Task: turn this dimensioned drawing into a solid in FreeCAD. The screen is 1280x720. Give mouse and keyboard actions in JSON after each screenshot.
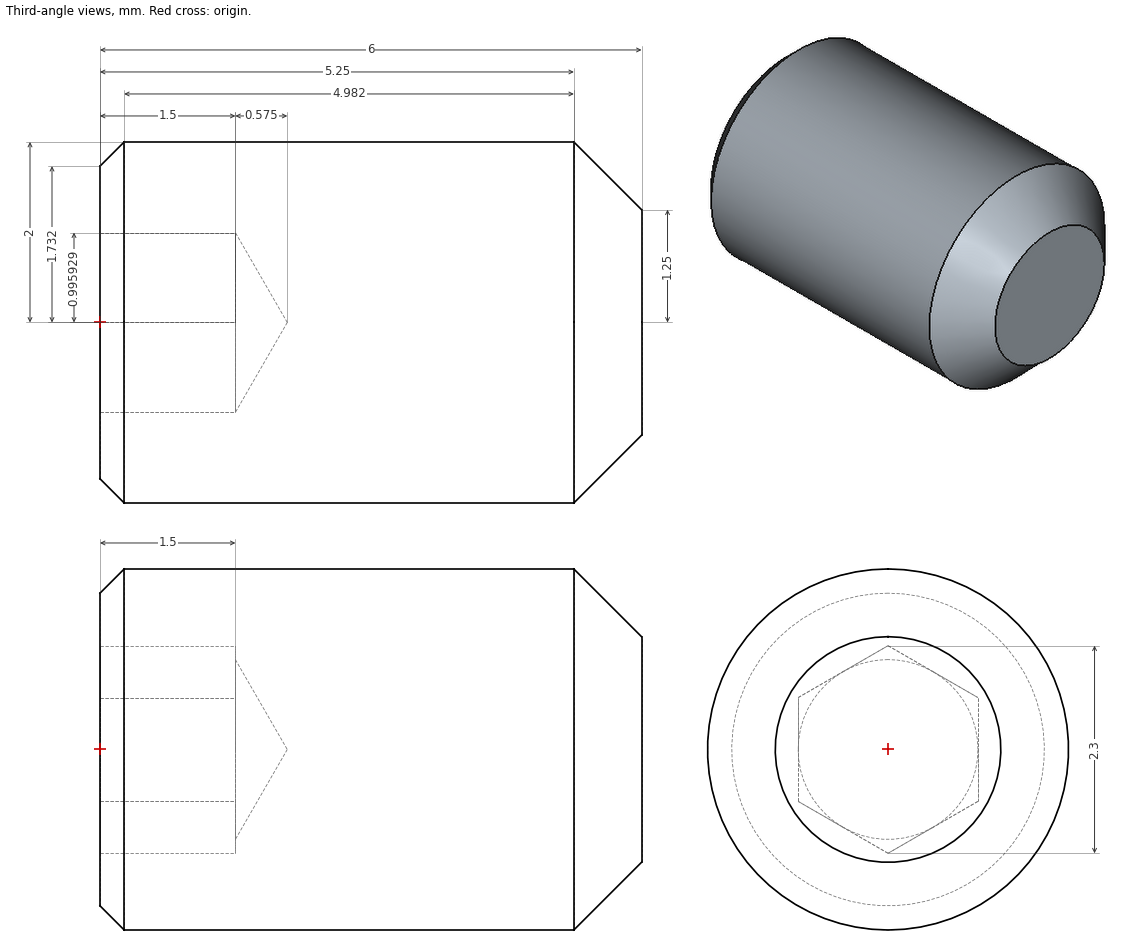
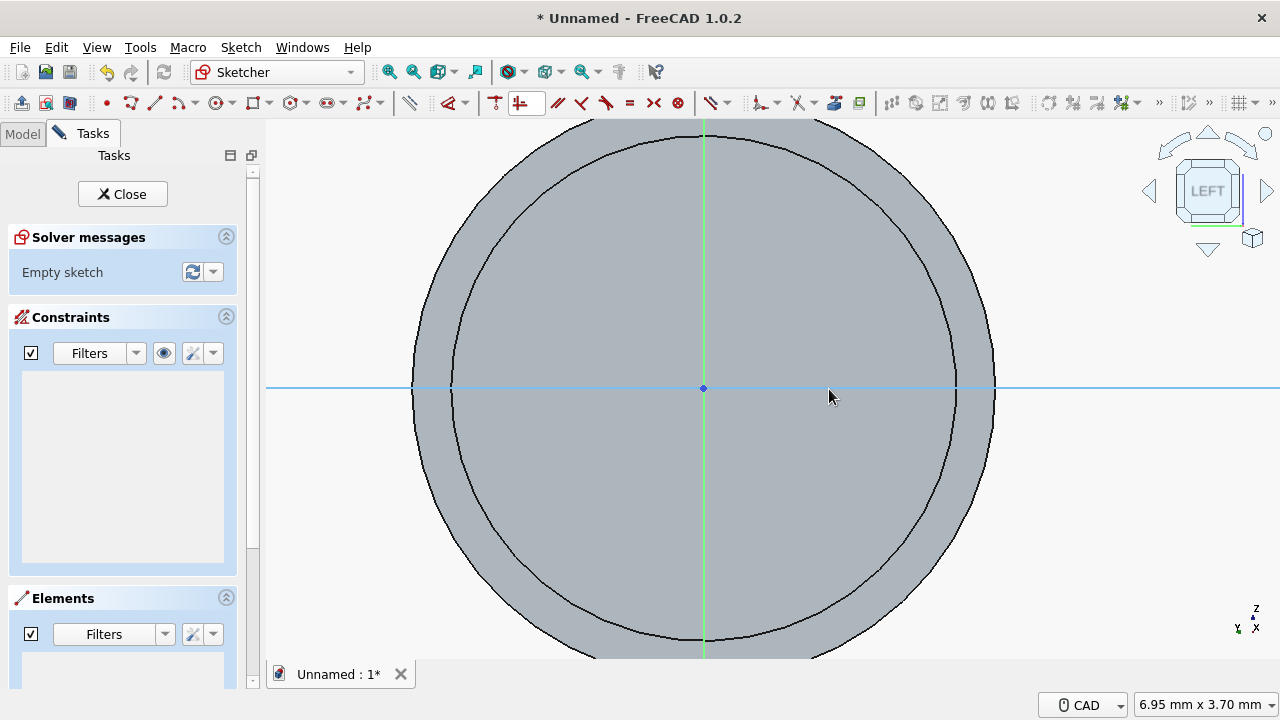
{"action": "left_click", "coordinate": [290, 104]}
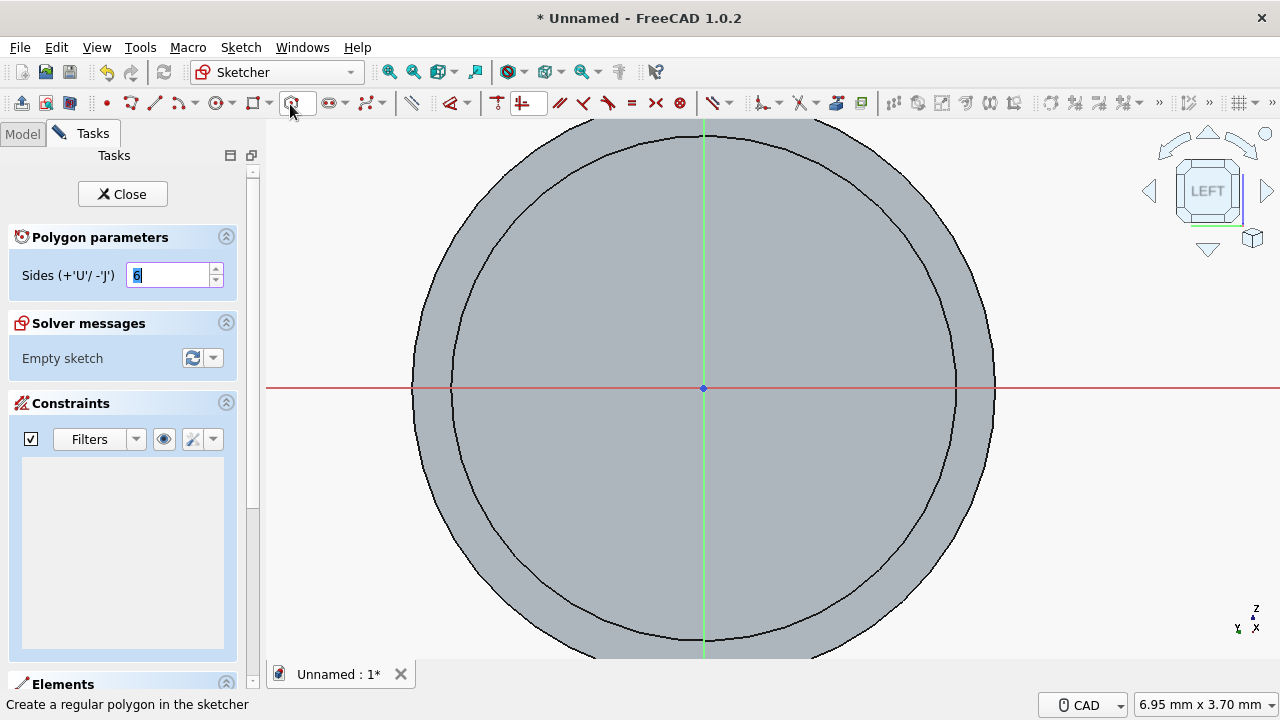
{"action": "left_click", "coordinate": [704, 388]}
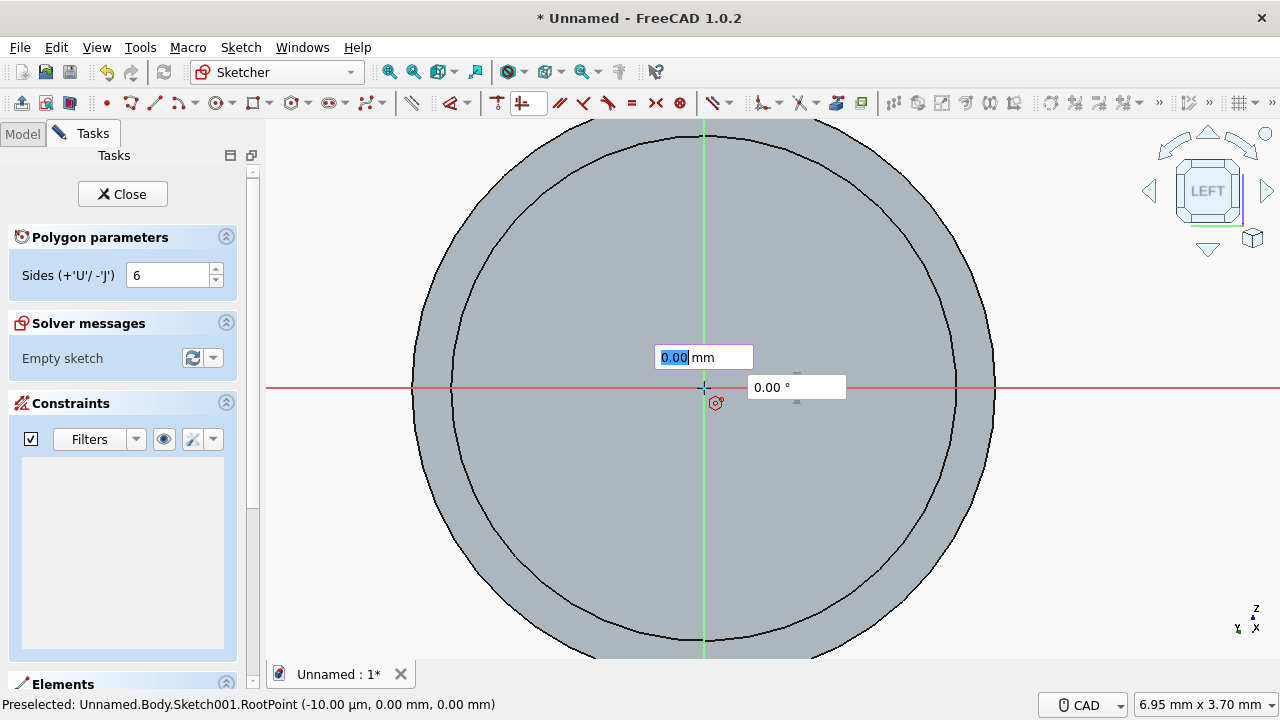
{"action": "left_click", "coordinate": [704, 221]}
{"action": "right_click", "coordinate": [704, 221]}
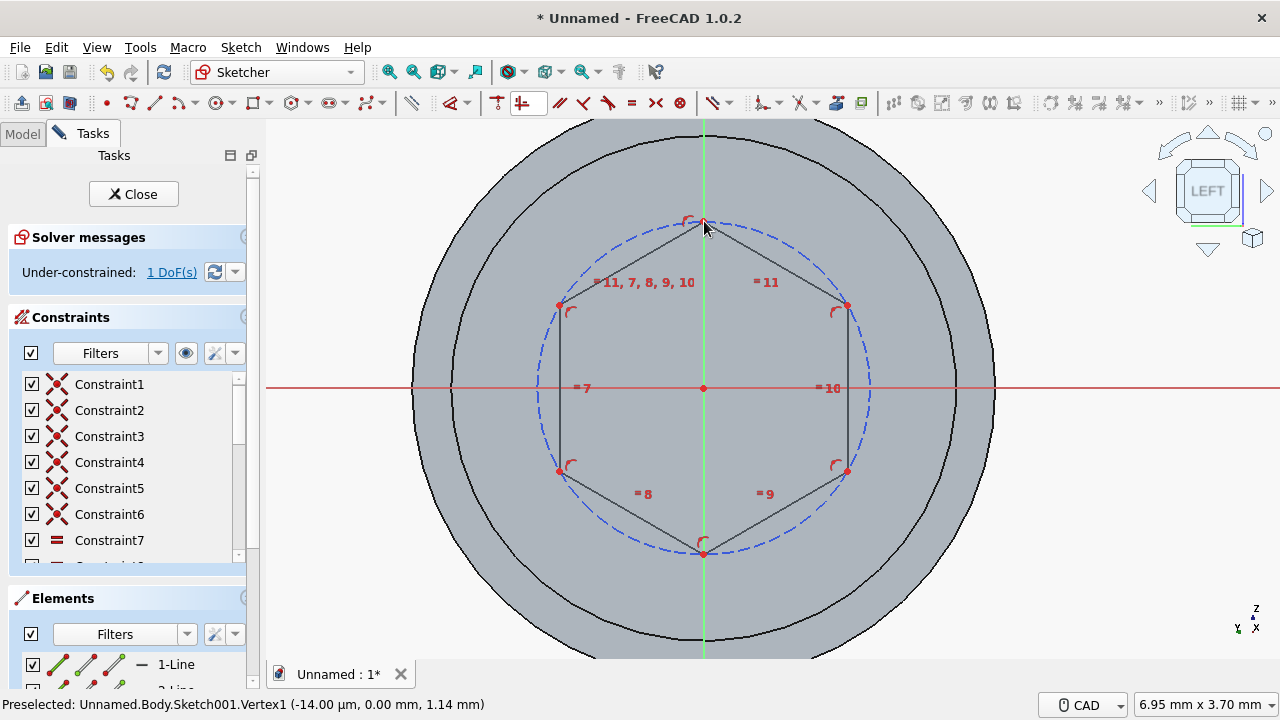
{"action": "left_click", "coordinate": [450, 104]}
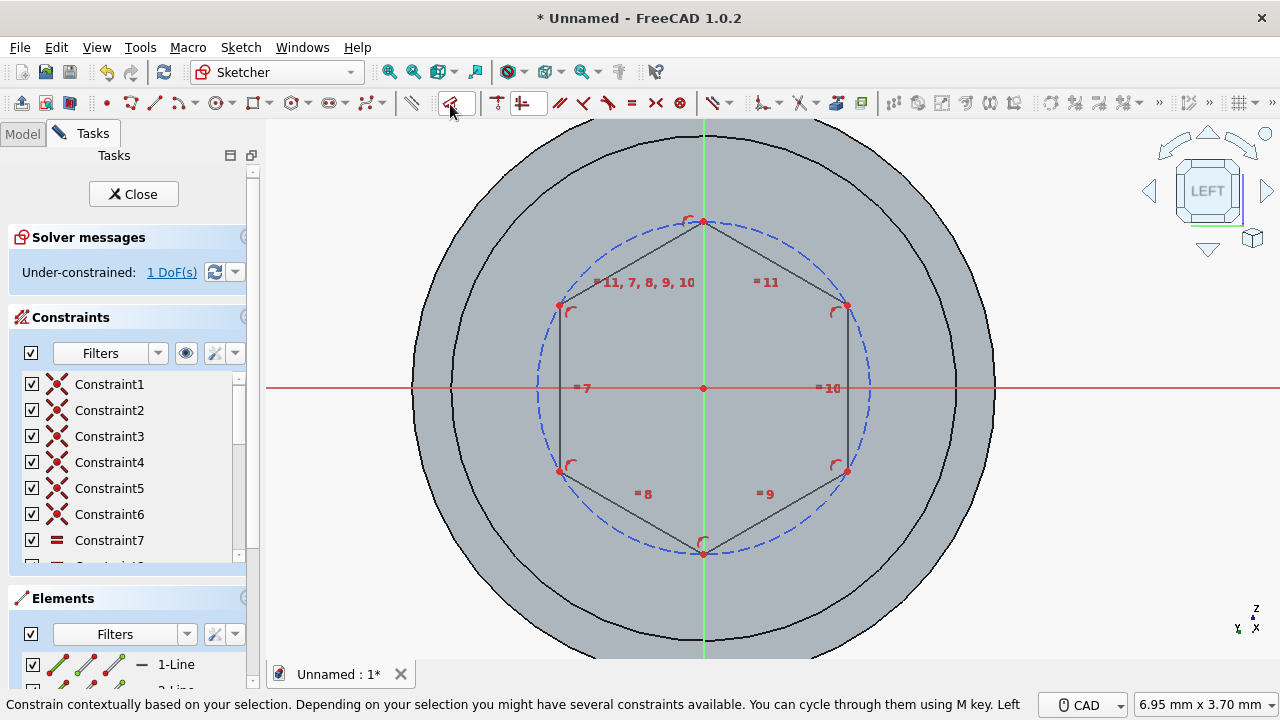
{"action": "left_click", "coordinate": [704, 555]}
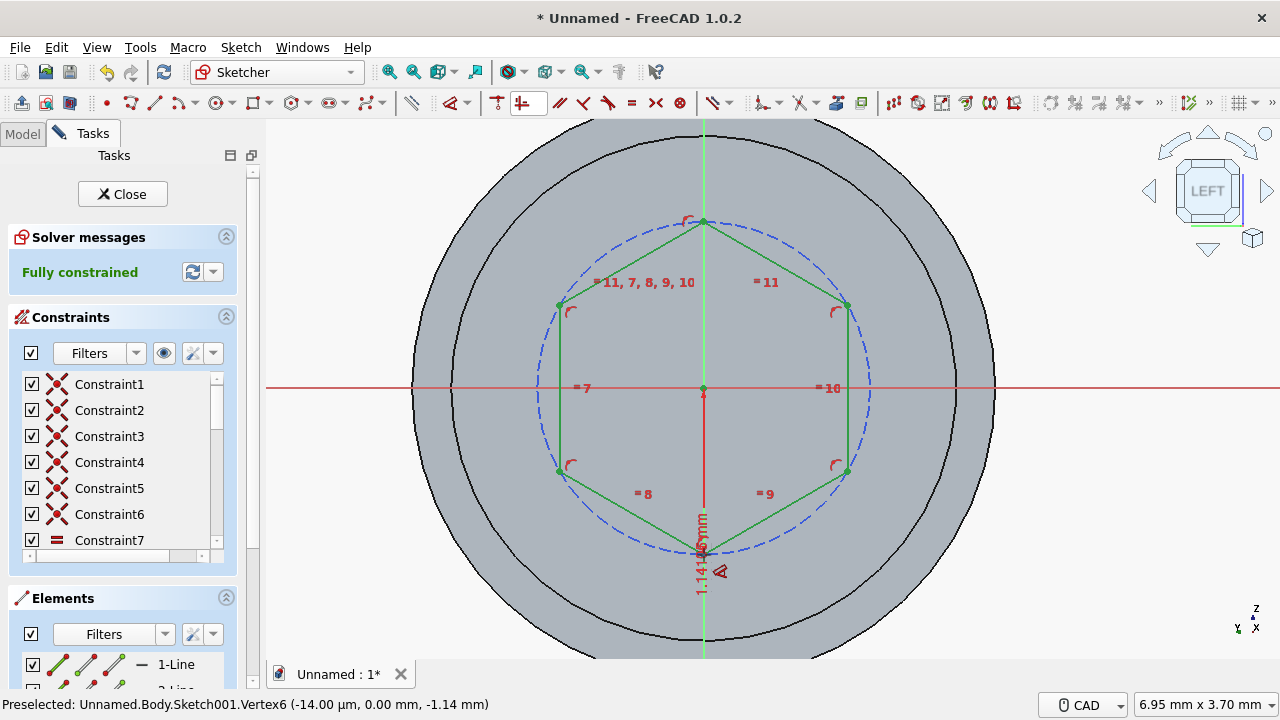
{"action": "left_click", "coordinate": [704, 222]}
{"action": "left_click", "coordinate": [738, 312]}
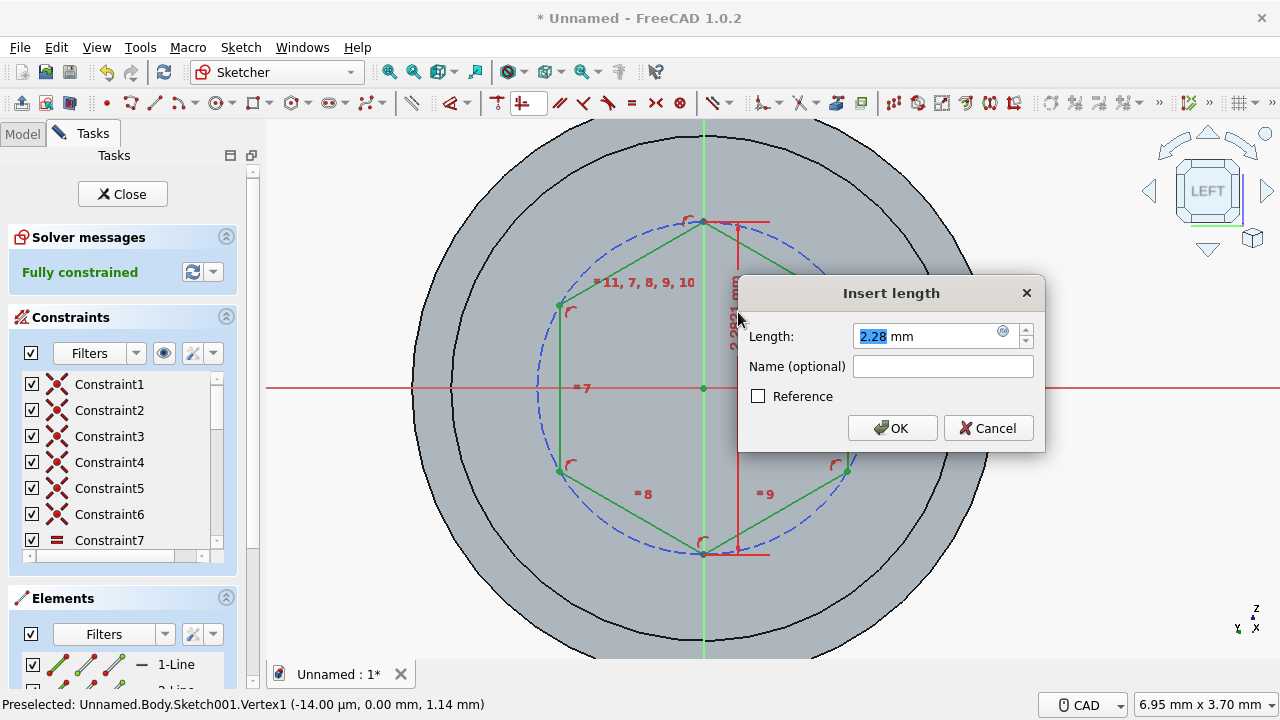
{"action": "type", "text": "2.3"}
{"action": "key", "text": "Return"}
{"action": "key", "text": "Escape"}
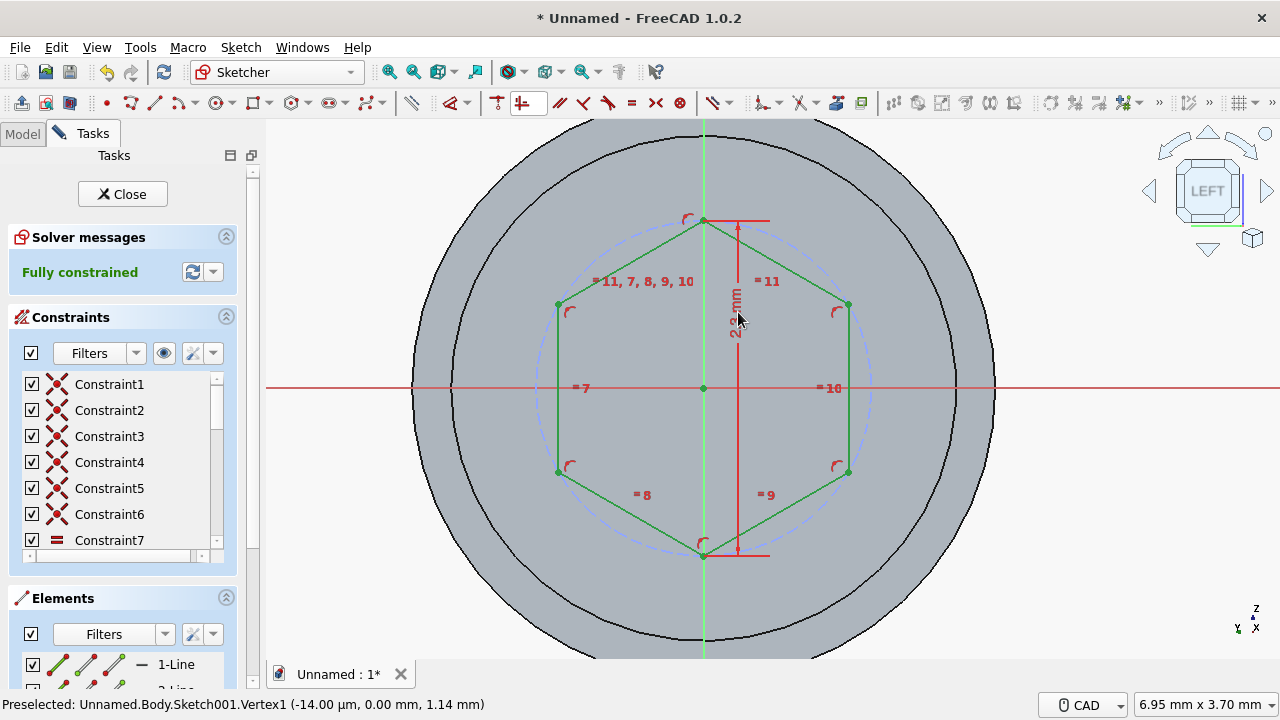
{"action": "left_click", "coordinate": [123, 194]}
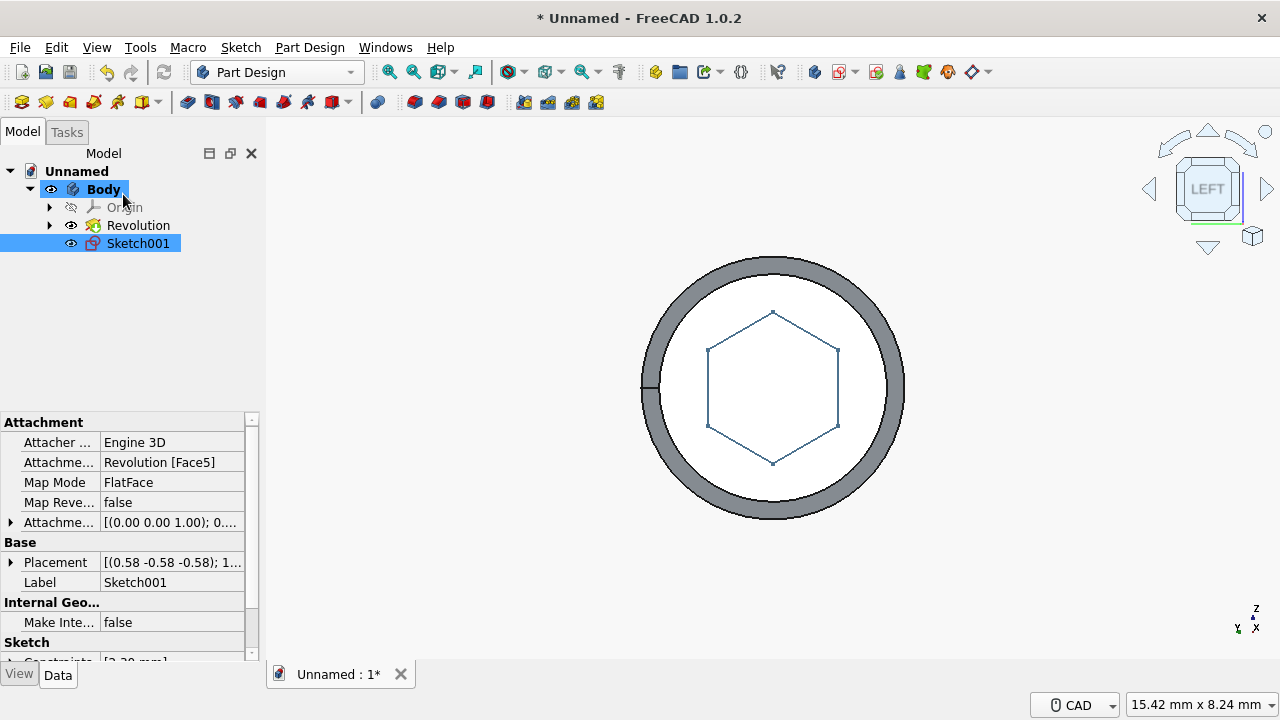
{"action": "left_click", "coordinate": [188, 102]}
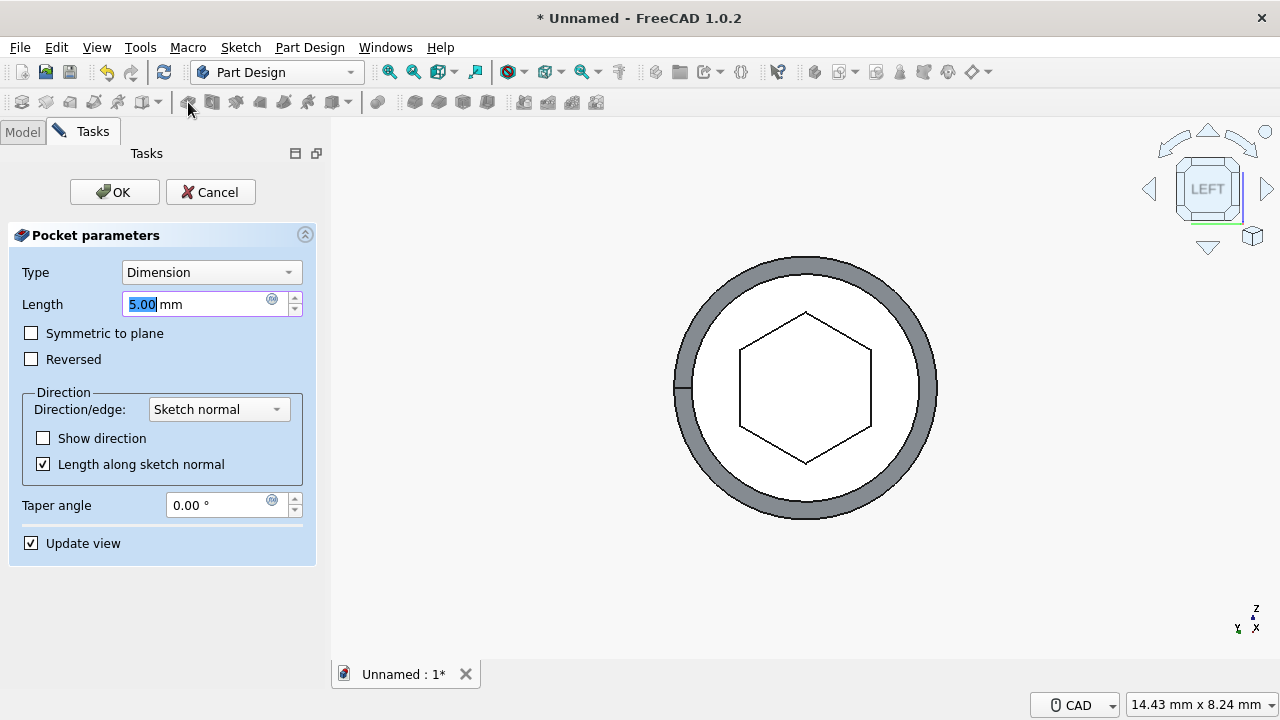
{"action": "type", "text": "1.5"}
{"action": "key", "text": "Tab"}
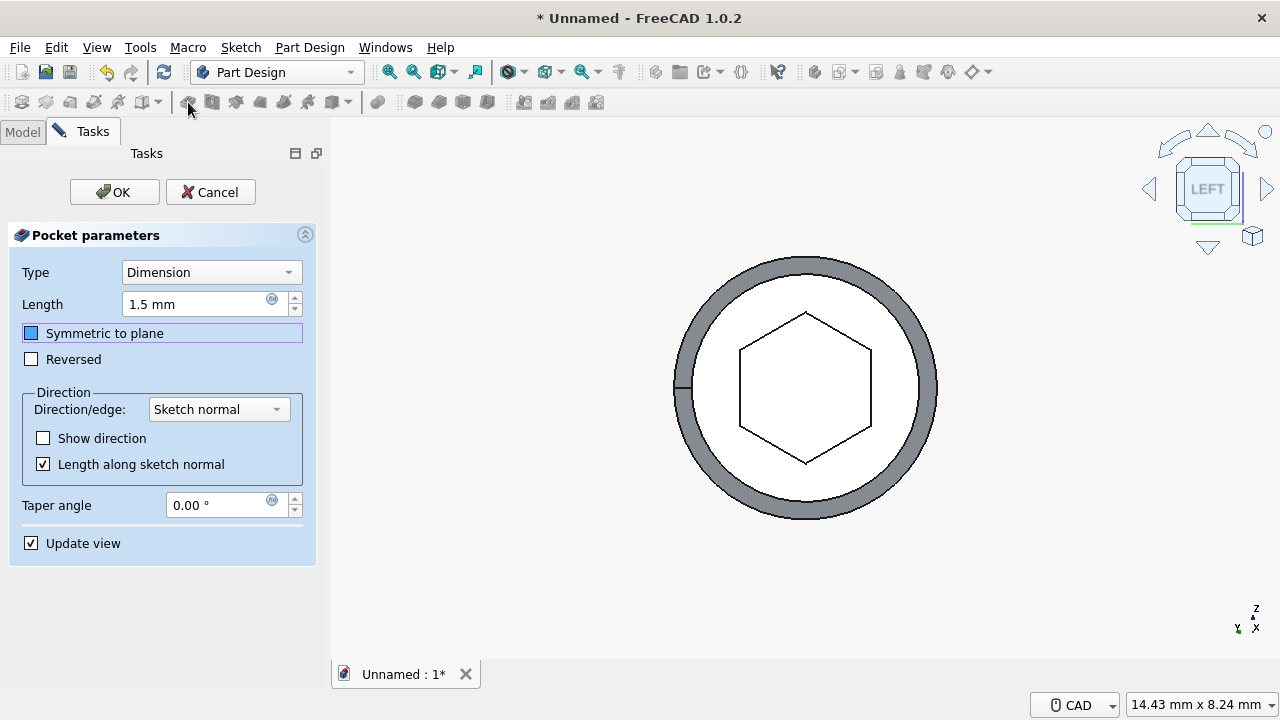
{"action": "left_click", "coordinate": [115, 192]}